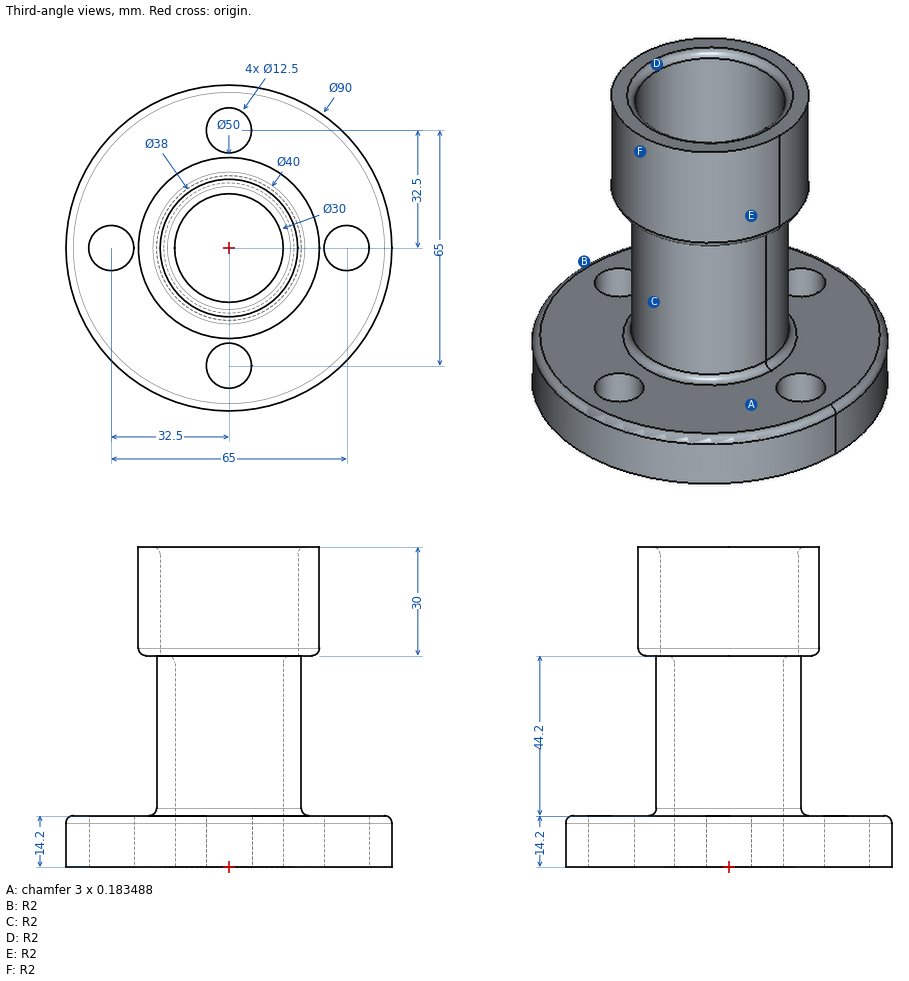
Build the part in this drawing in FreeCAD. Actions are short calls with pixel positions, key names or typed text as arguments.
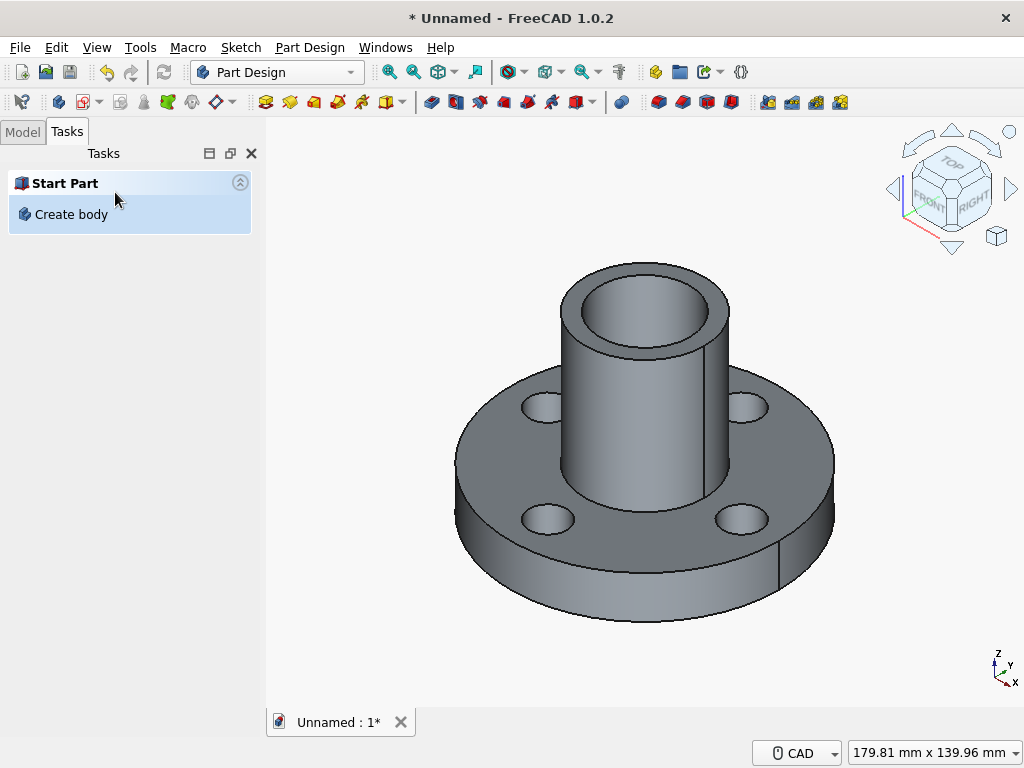
key(2)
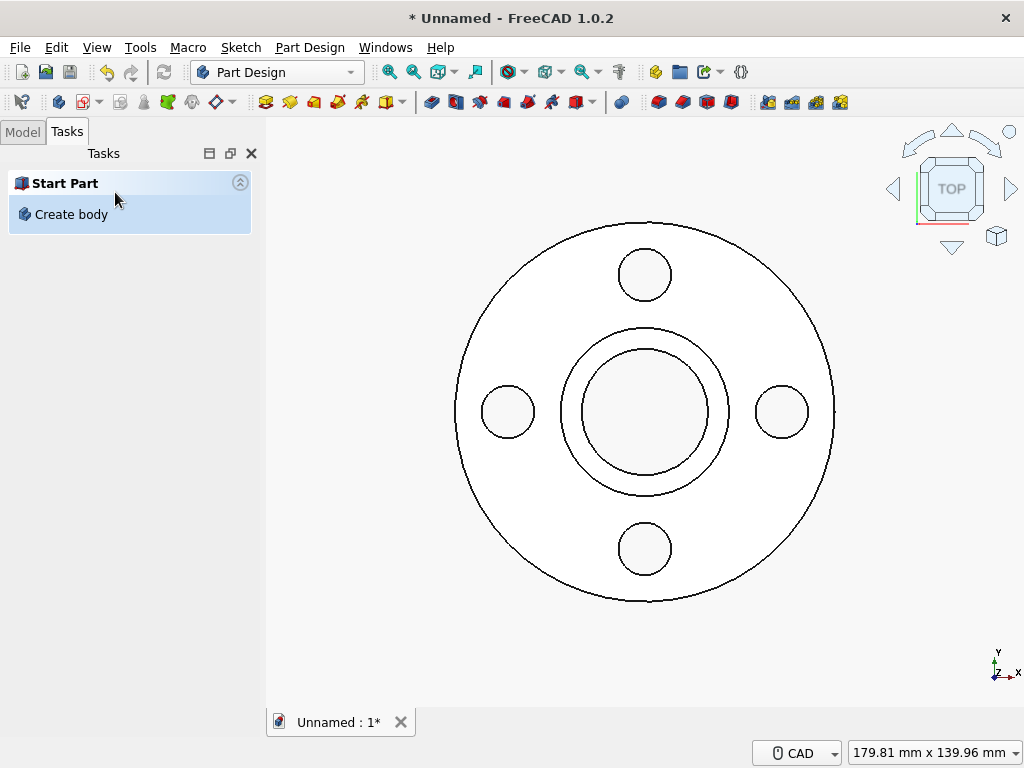
key(1)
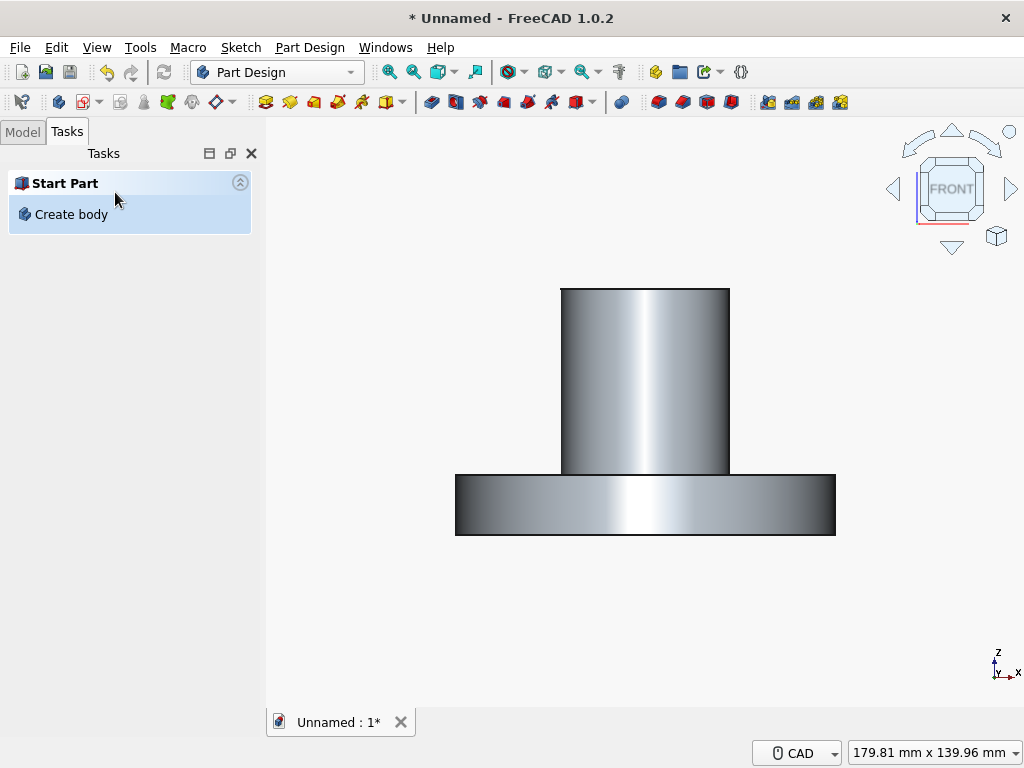
key(3)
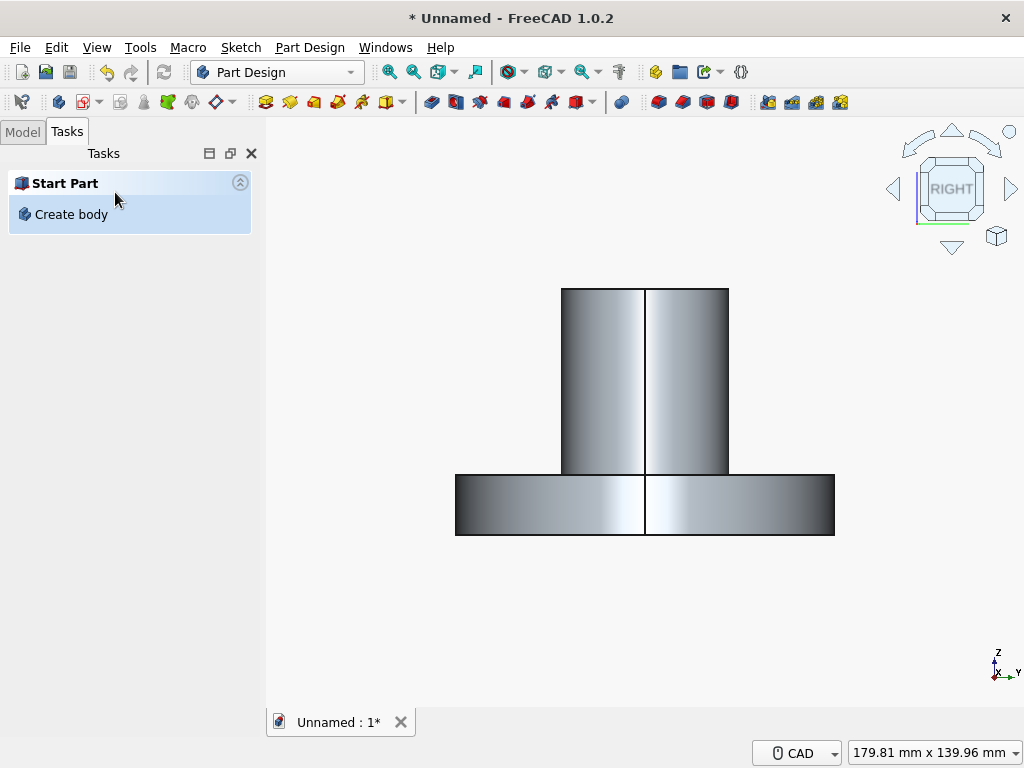
key(5)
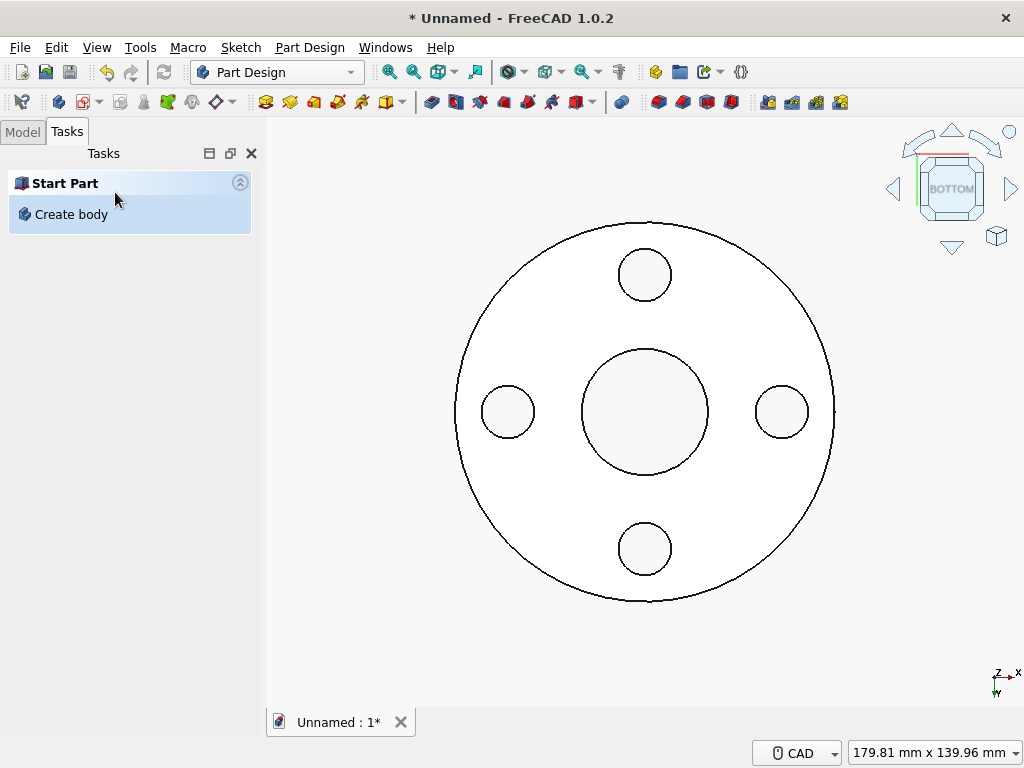
click(582, 411)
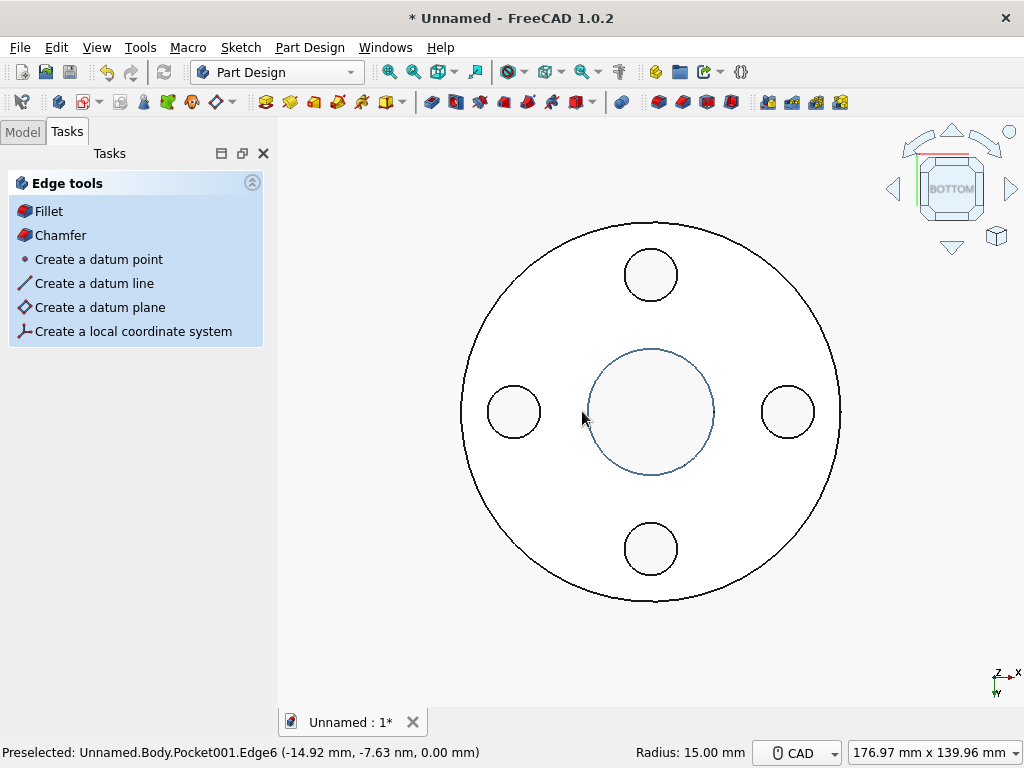
click(684, 102)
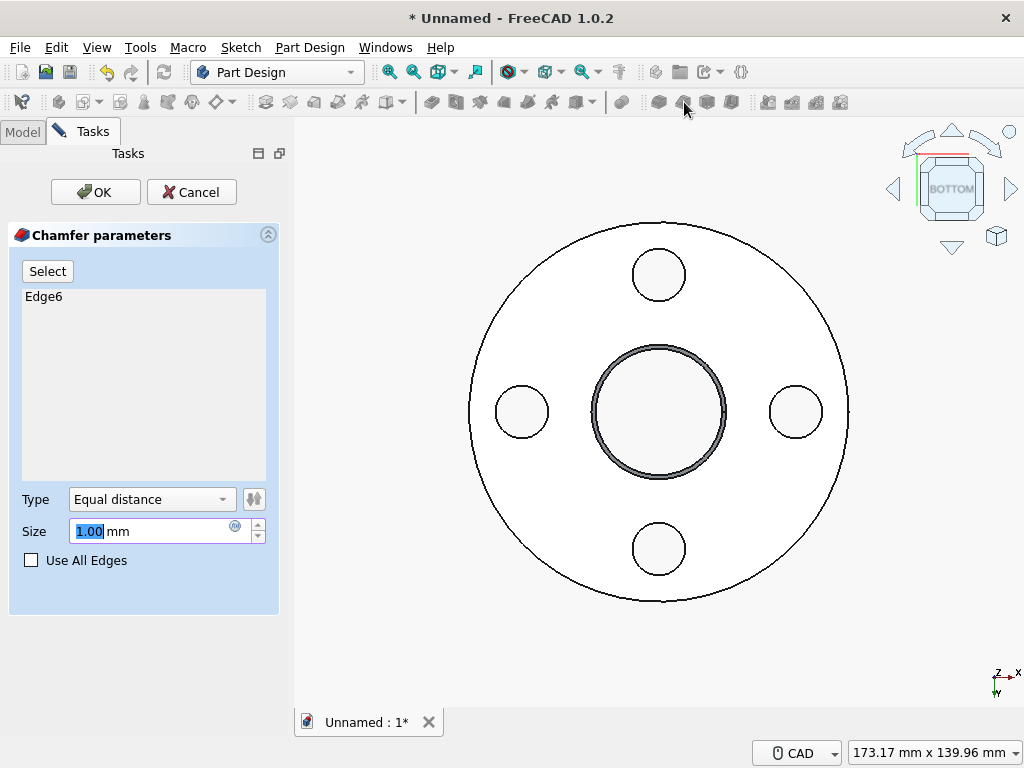
text(3)
key(Tab)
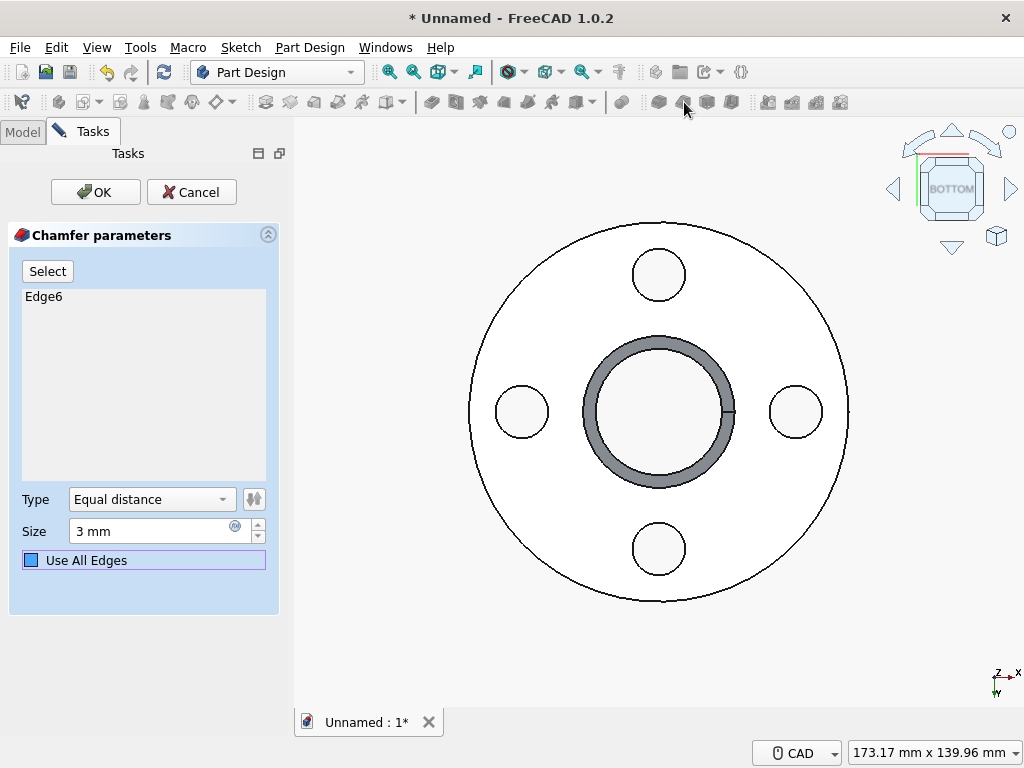
click(153, 500)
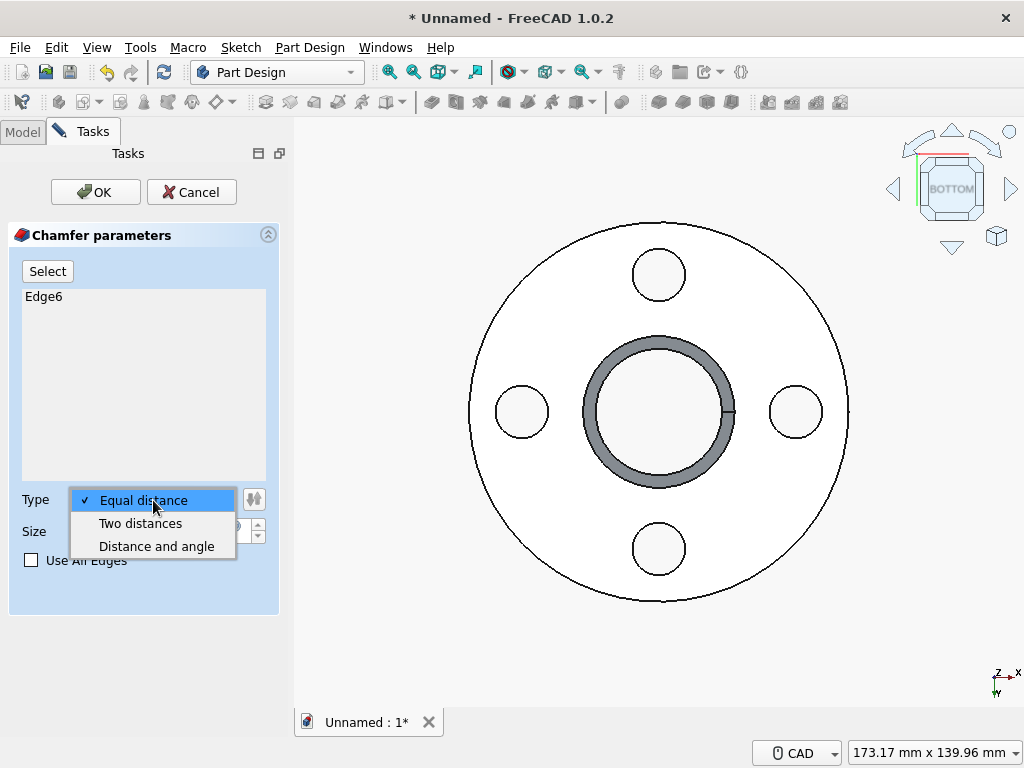
click(152, 524)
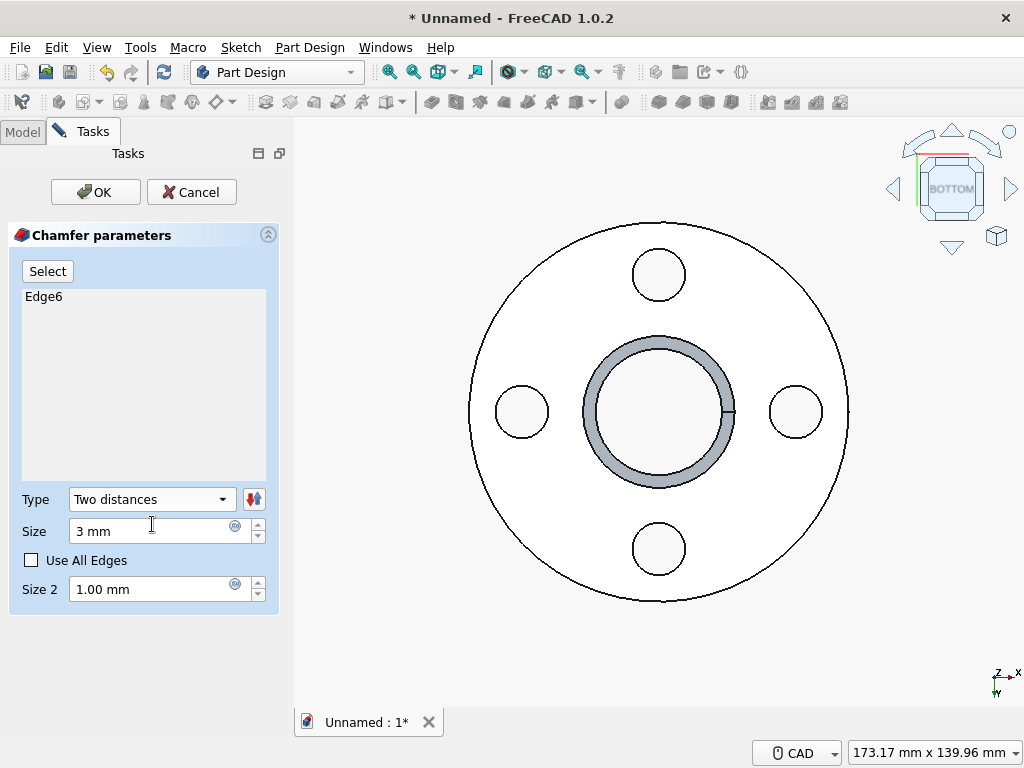
triple_click(160, 589)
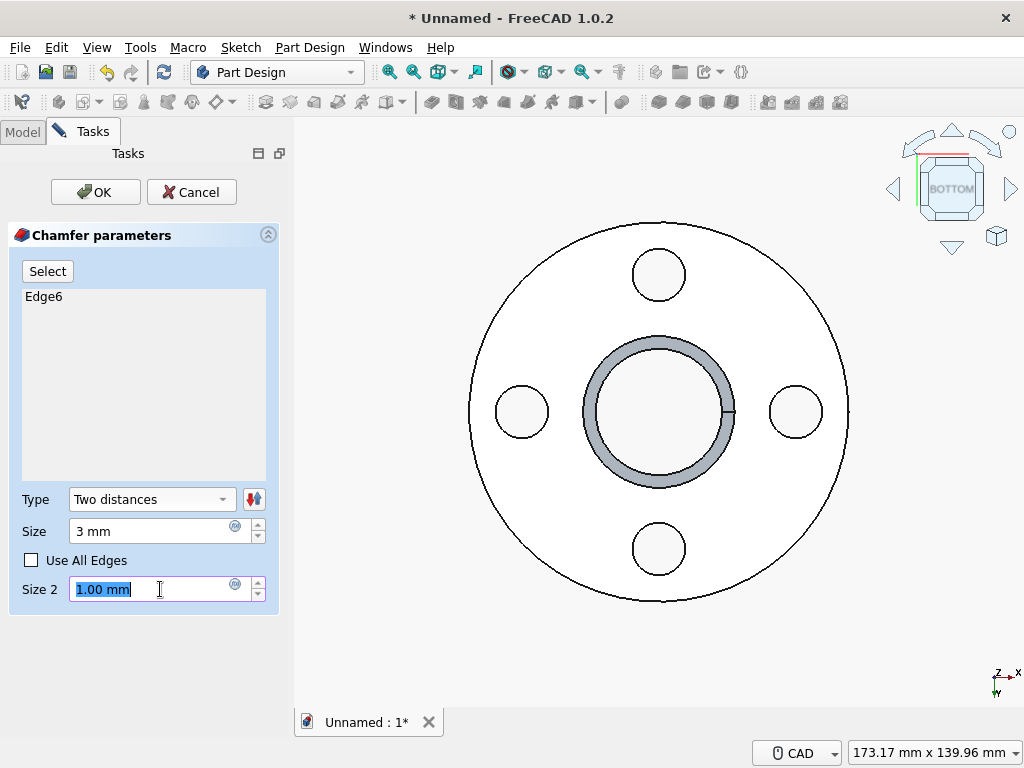
text(0.183488)
key(Tab)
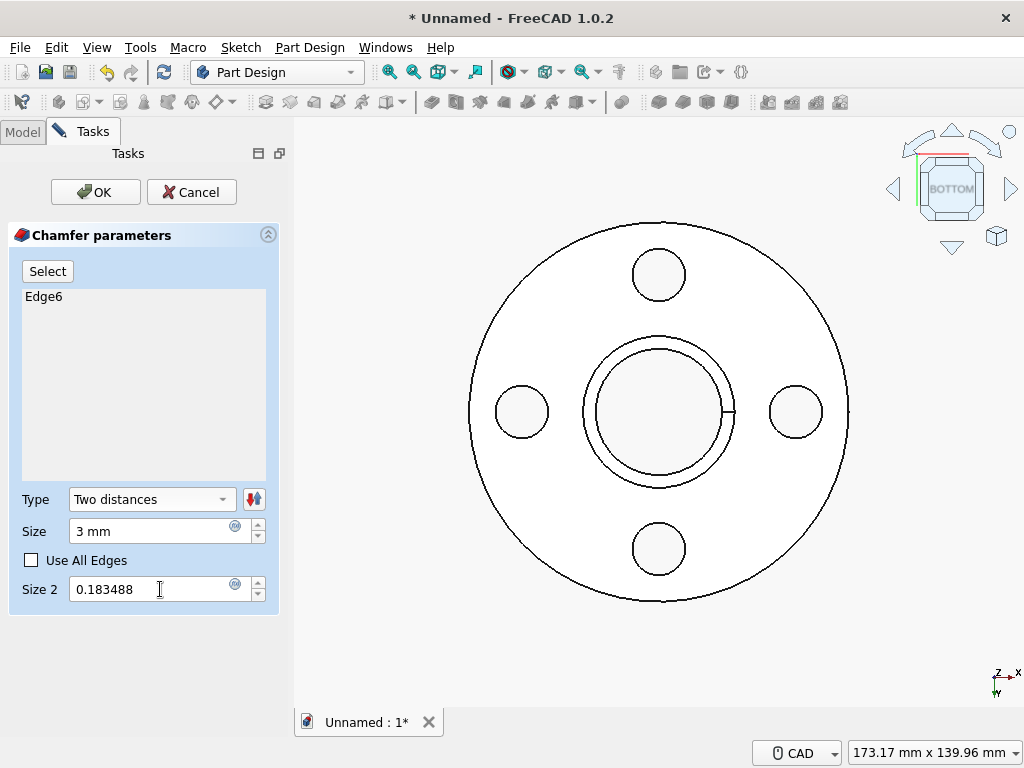
click(96, 192)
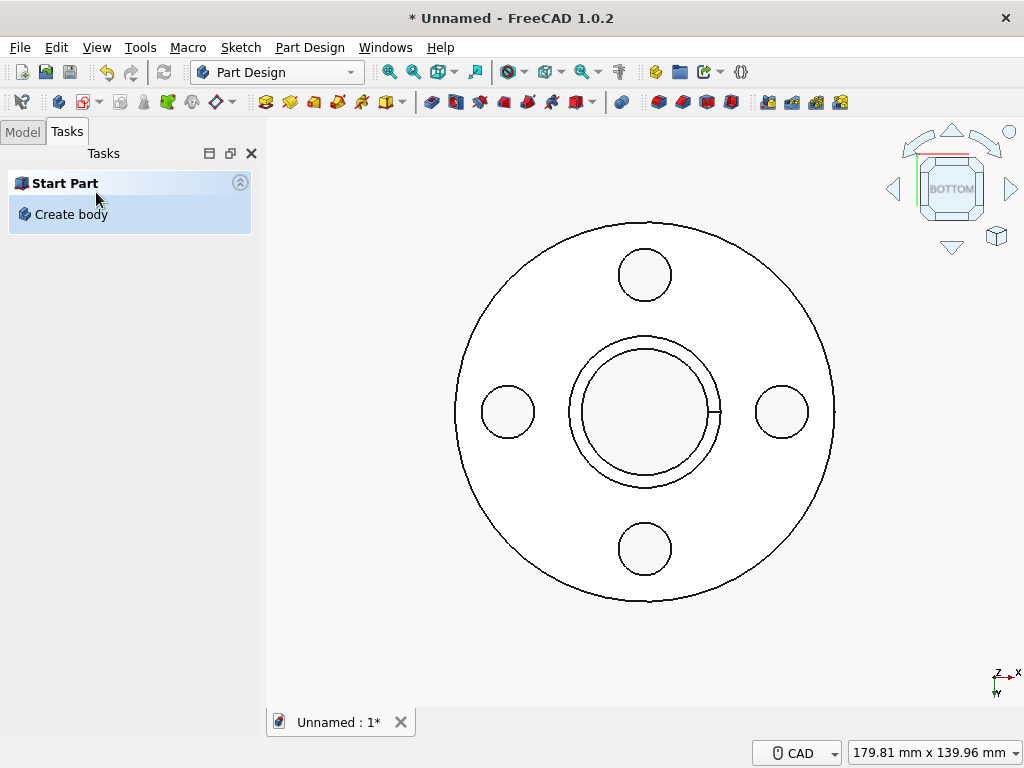
key(0)